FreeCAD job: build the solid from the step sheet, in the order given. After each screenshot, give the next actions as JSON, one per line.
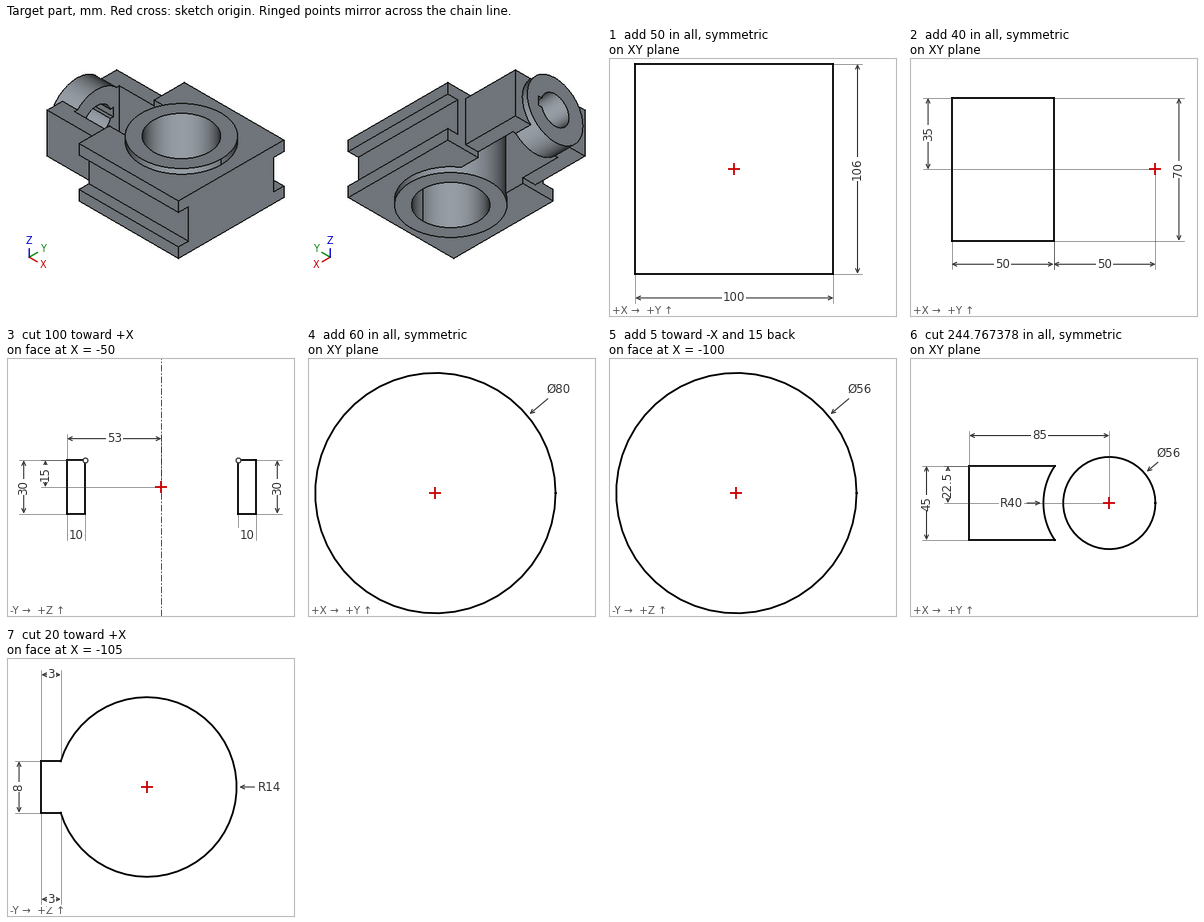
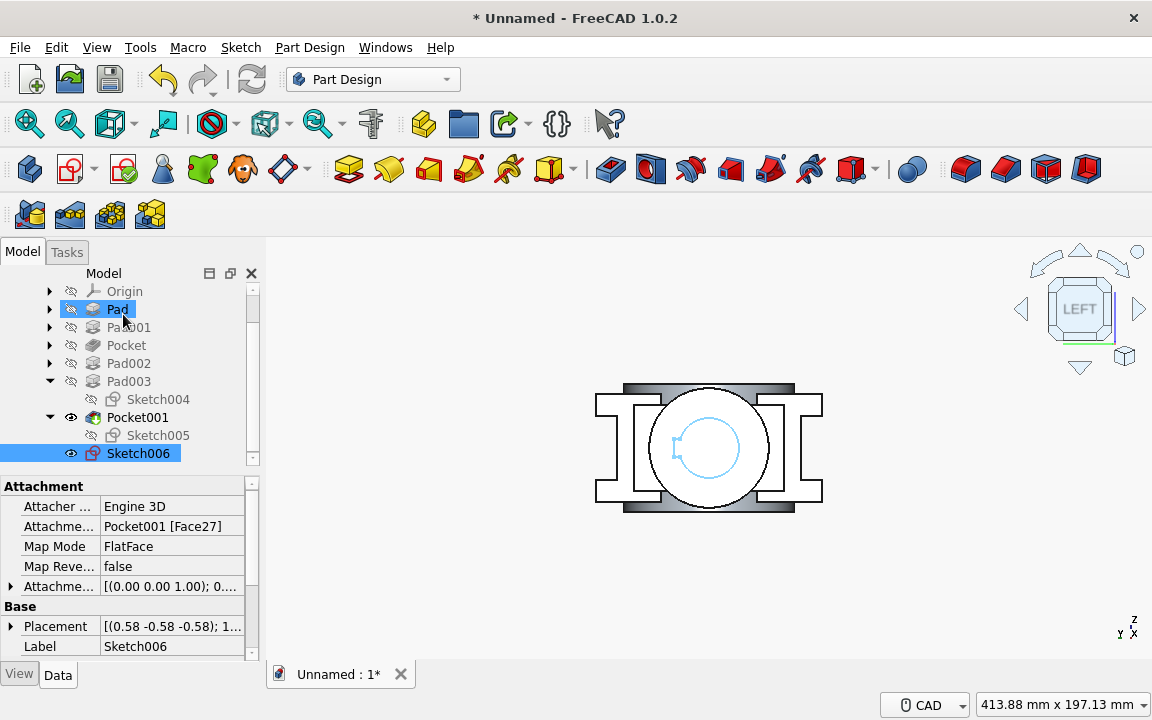
{"action": "left_click", "coordinate": [612, 170]}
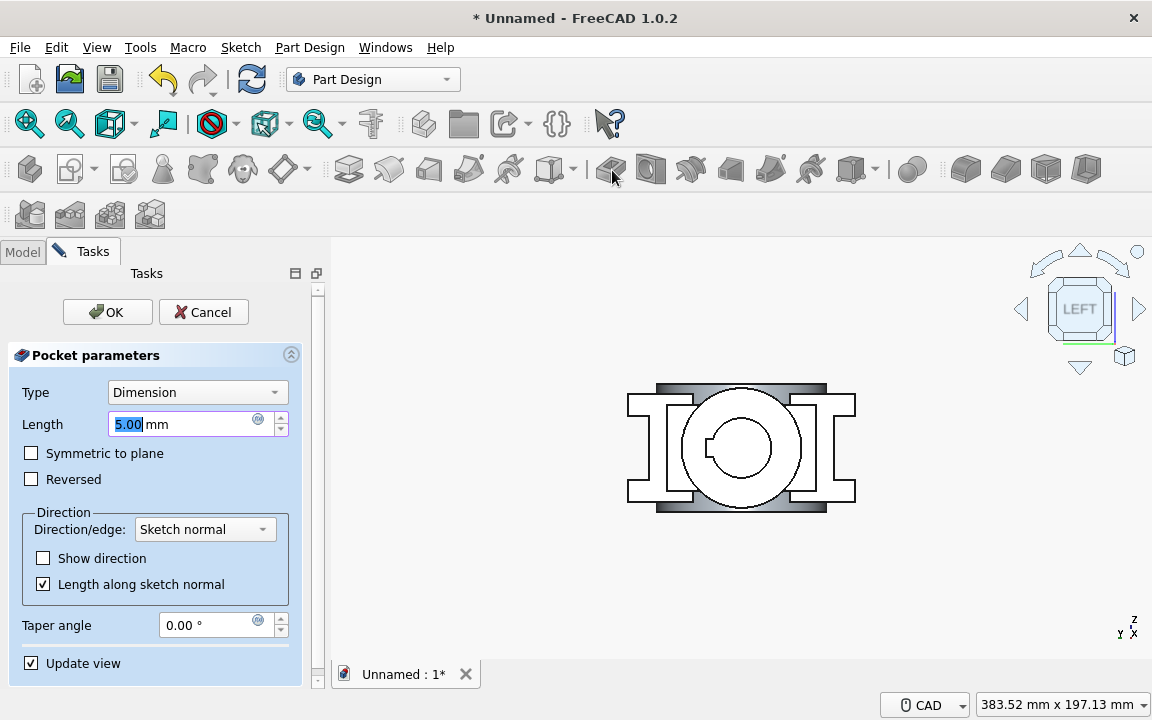
{"action": "type", "text": "20"}
{"action": "key", "text": "Tab"}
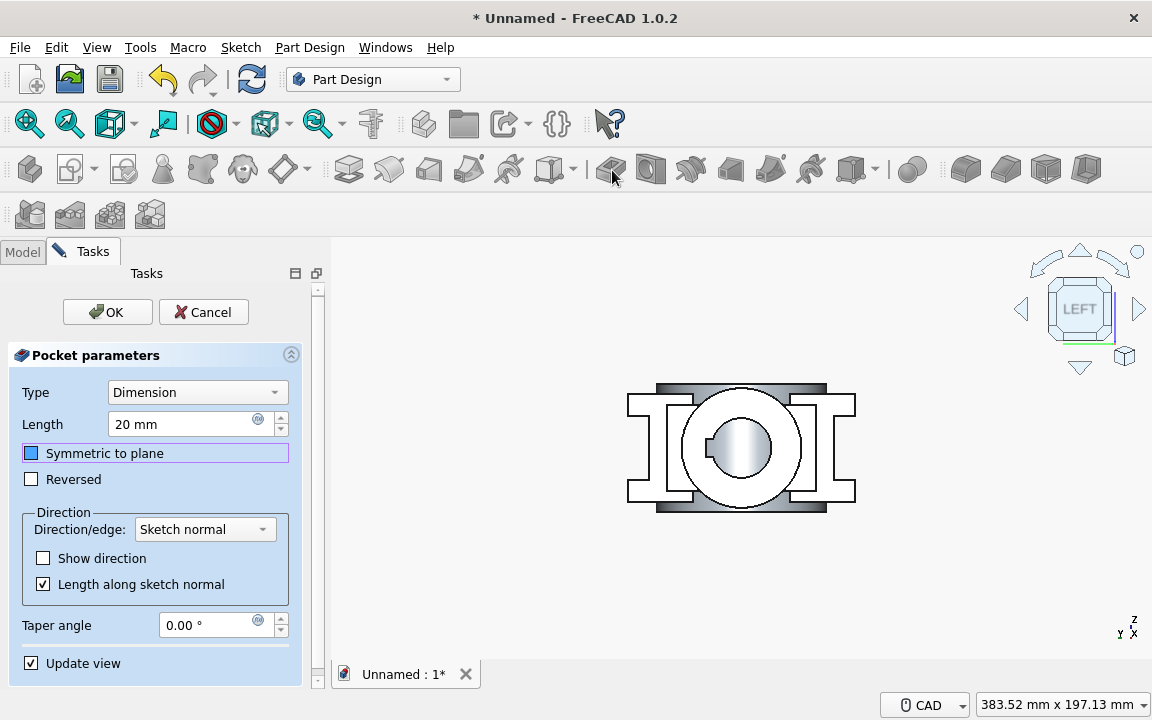
{"action": "left_click", "coordinate": [108, 312]}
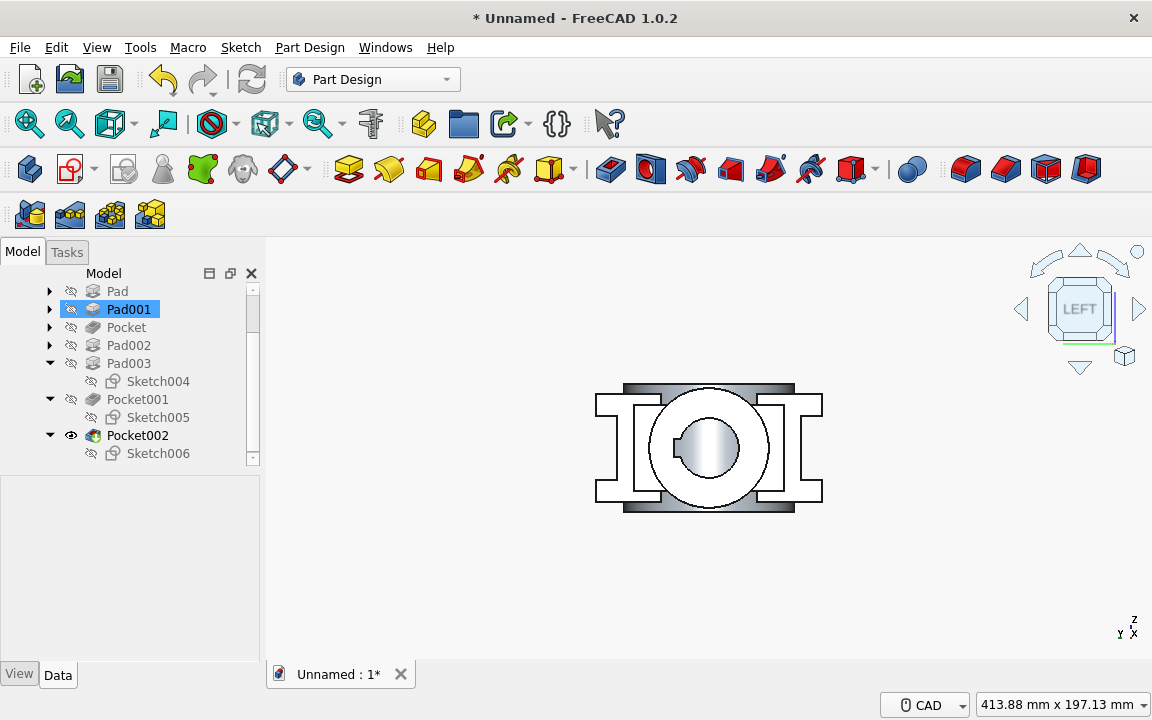
{"action": "key", "text": "0"}